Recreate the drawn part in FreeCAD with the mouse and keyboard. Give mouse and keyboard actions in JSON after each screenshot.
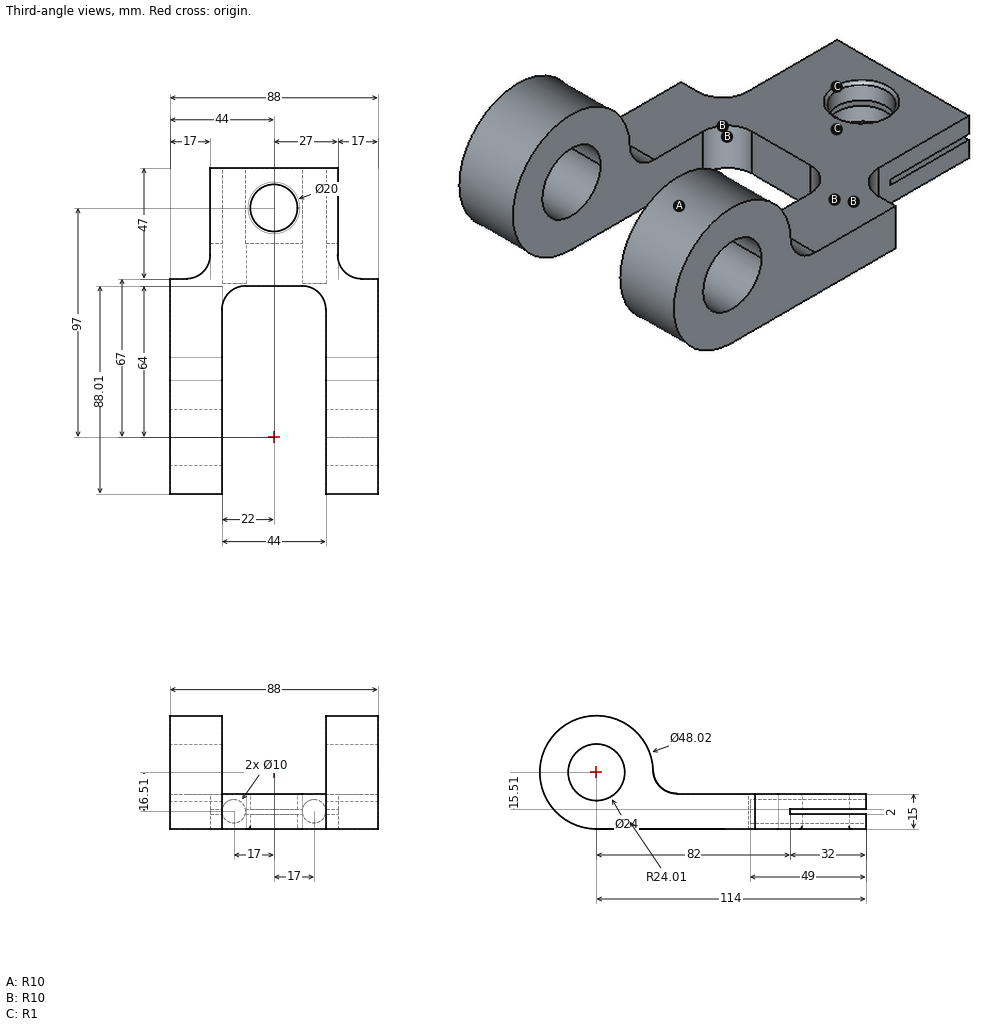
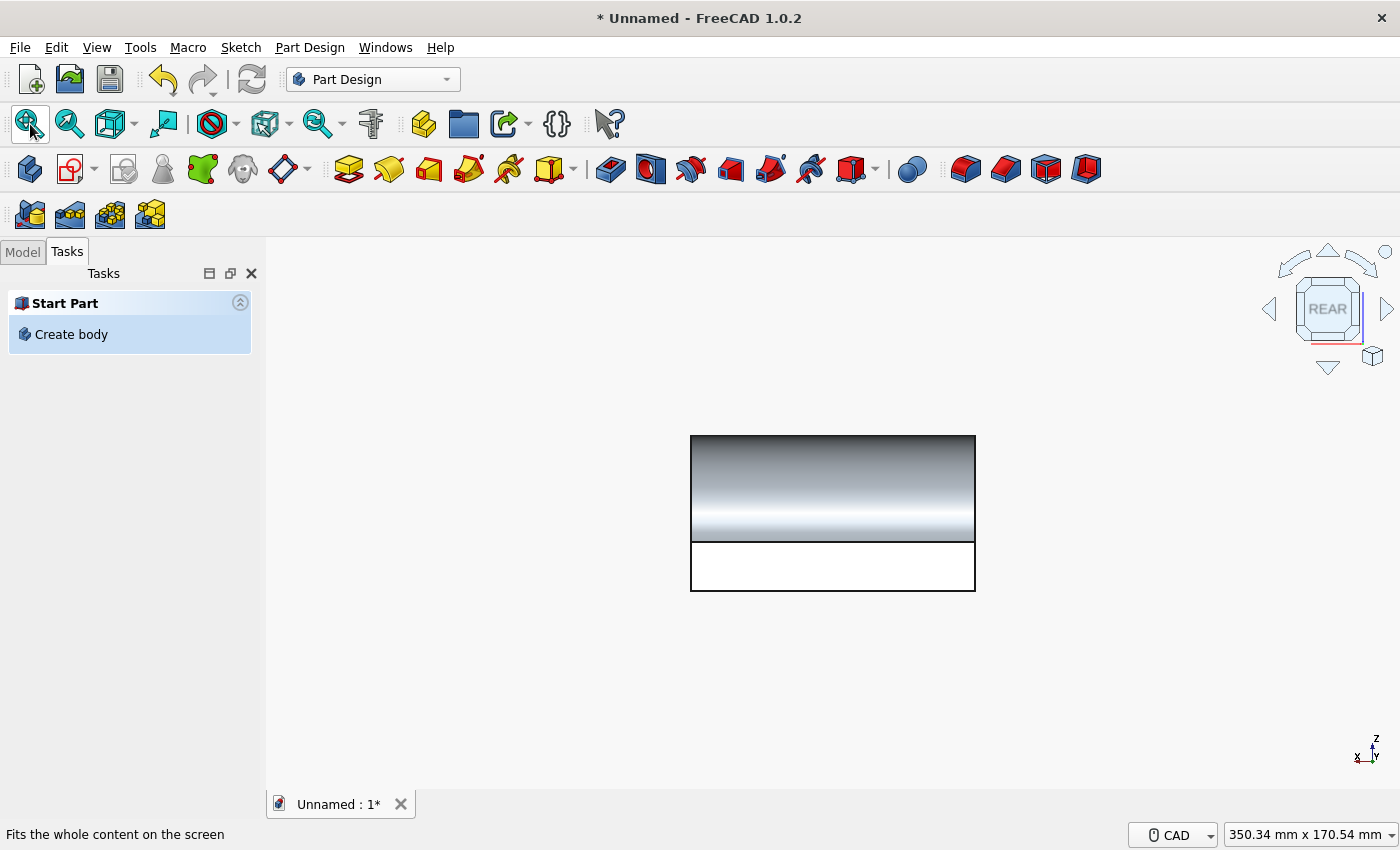
{"action": "key", "text": "6"}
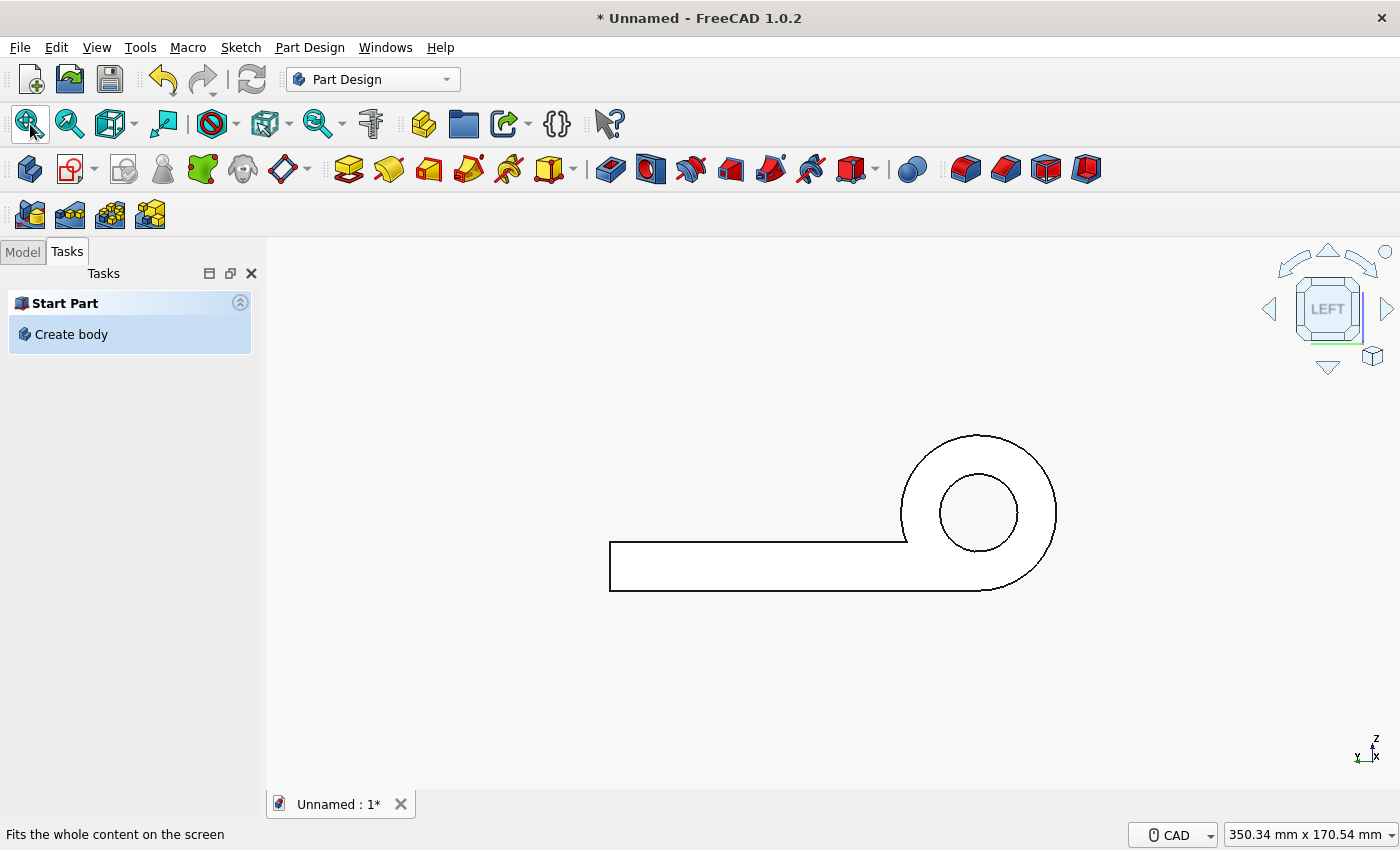
{"action": "left_click", "coordinate": [30, 124]}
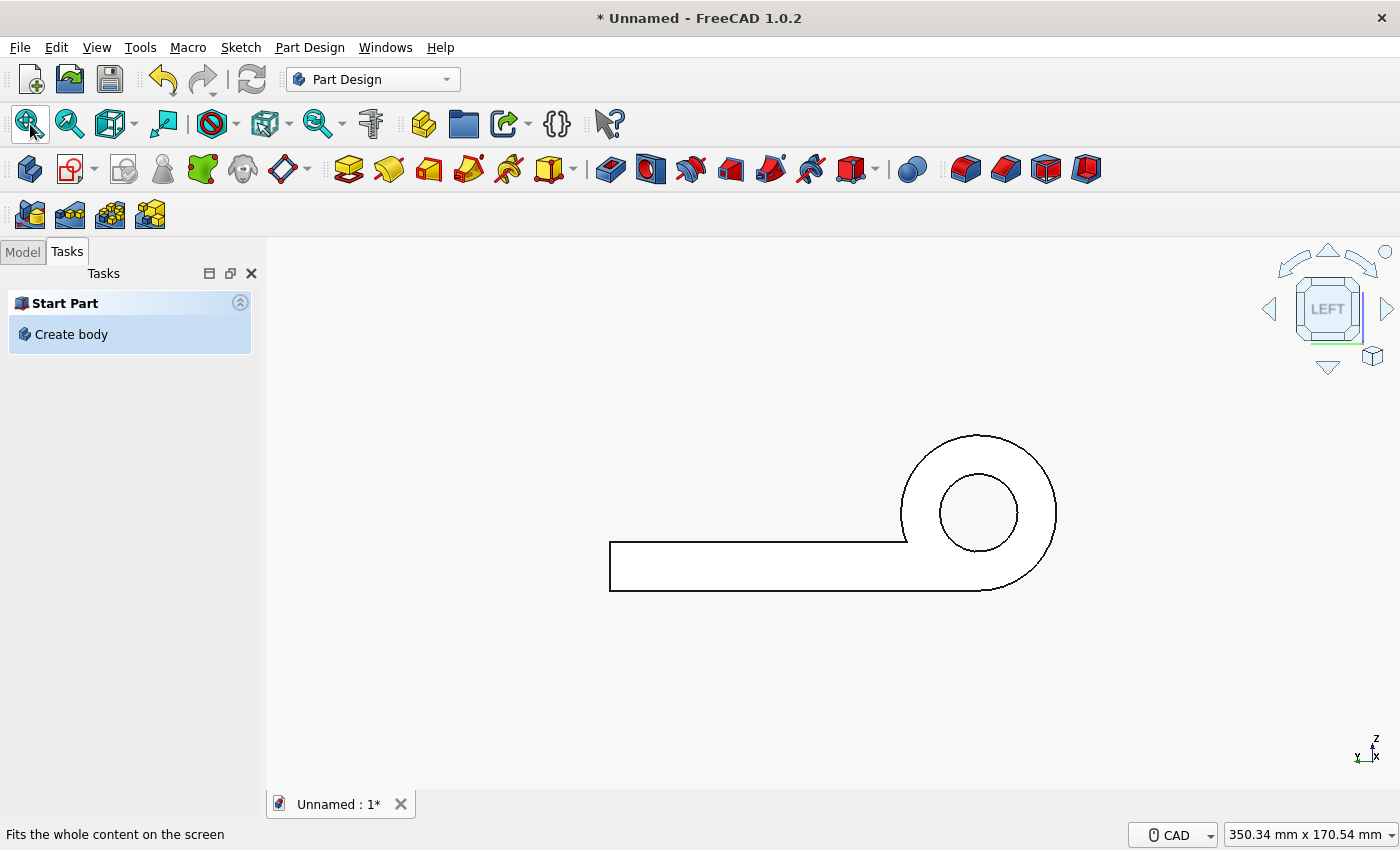
{"action": "key", "text": "v 3"}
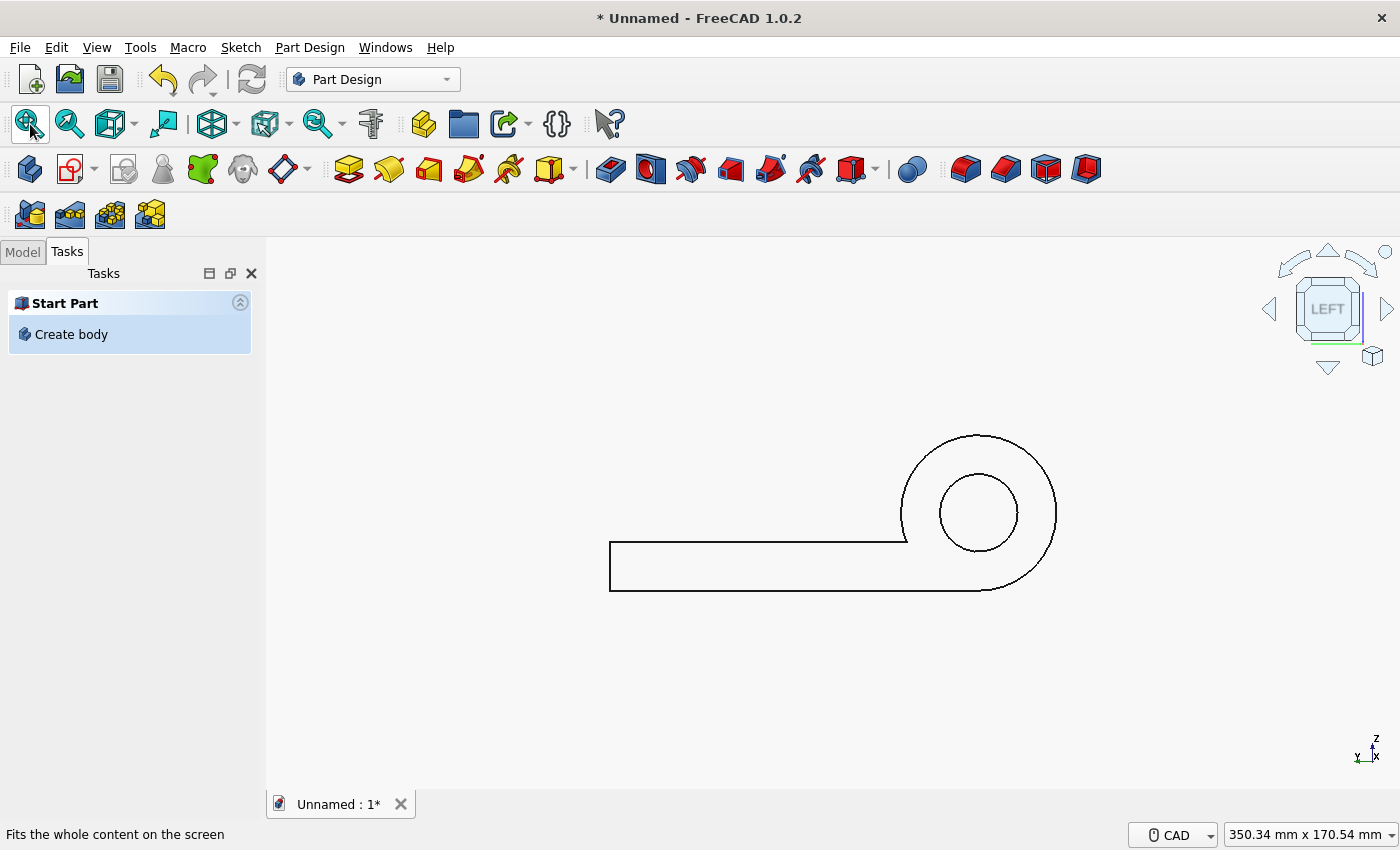
{"action": "key", "text": "0"}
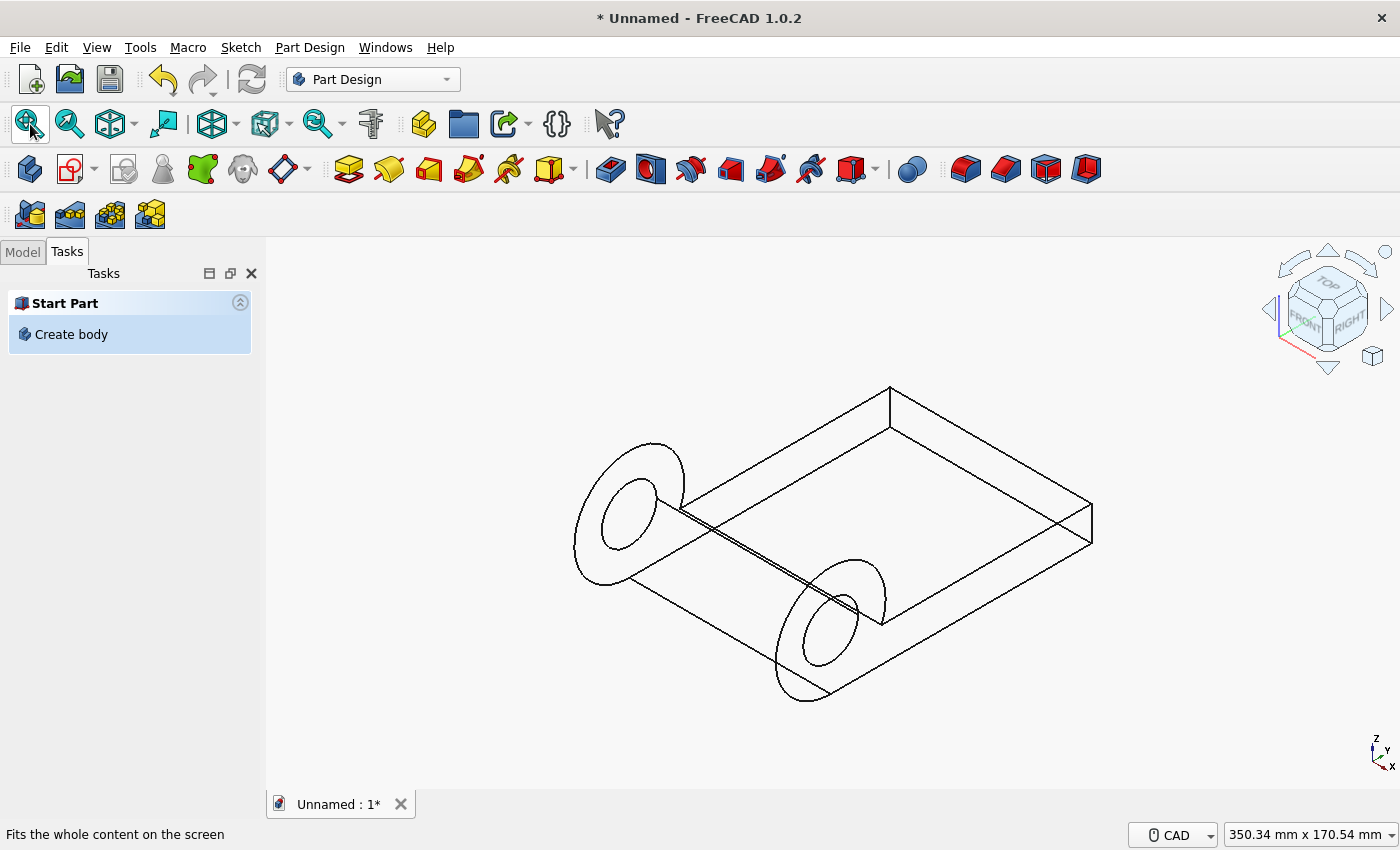
{"action": "key", "text": "2"}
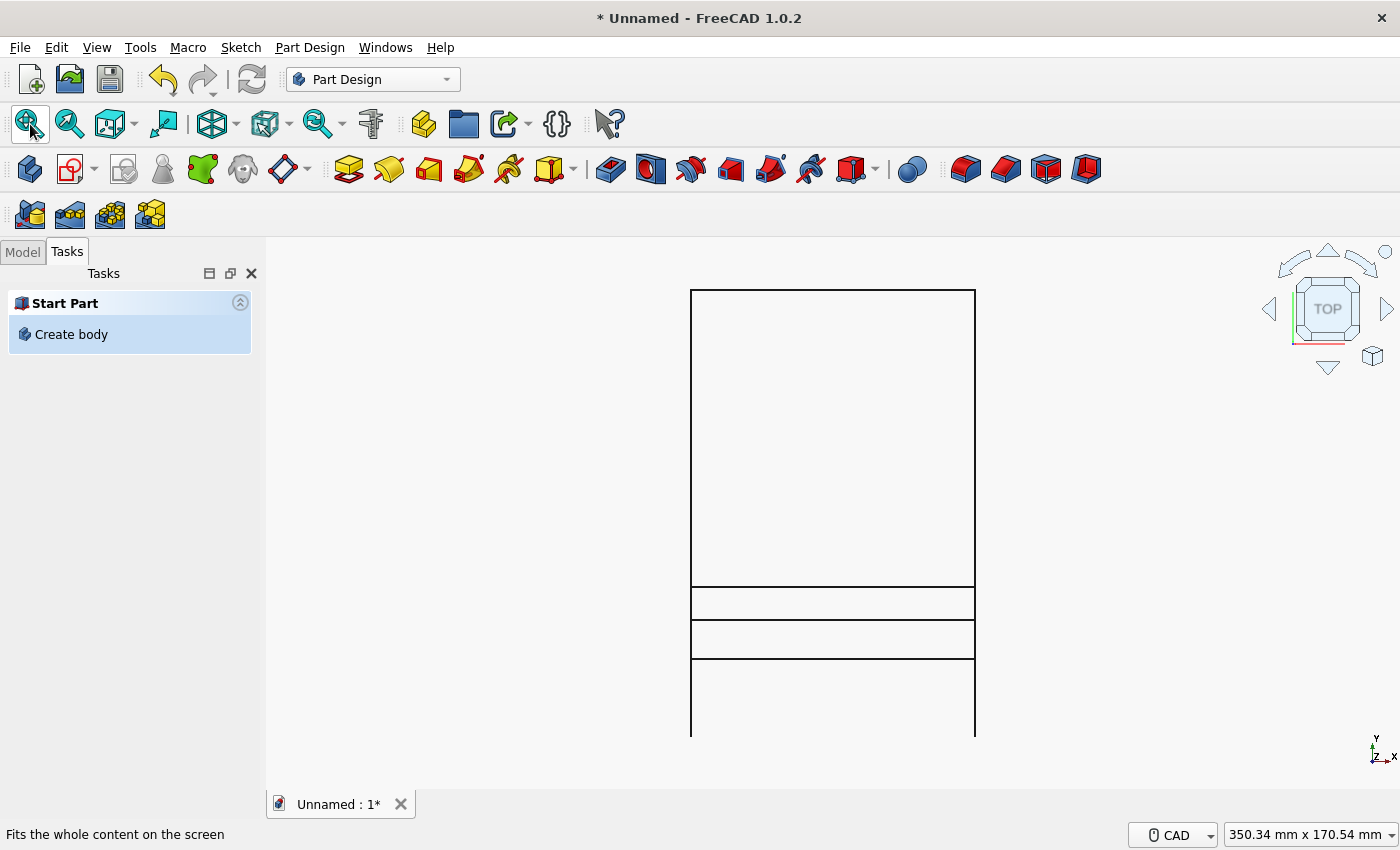
{"action": "left_click", "coordinate": [833, 586]}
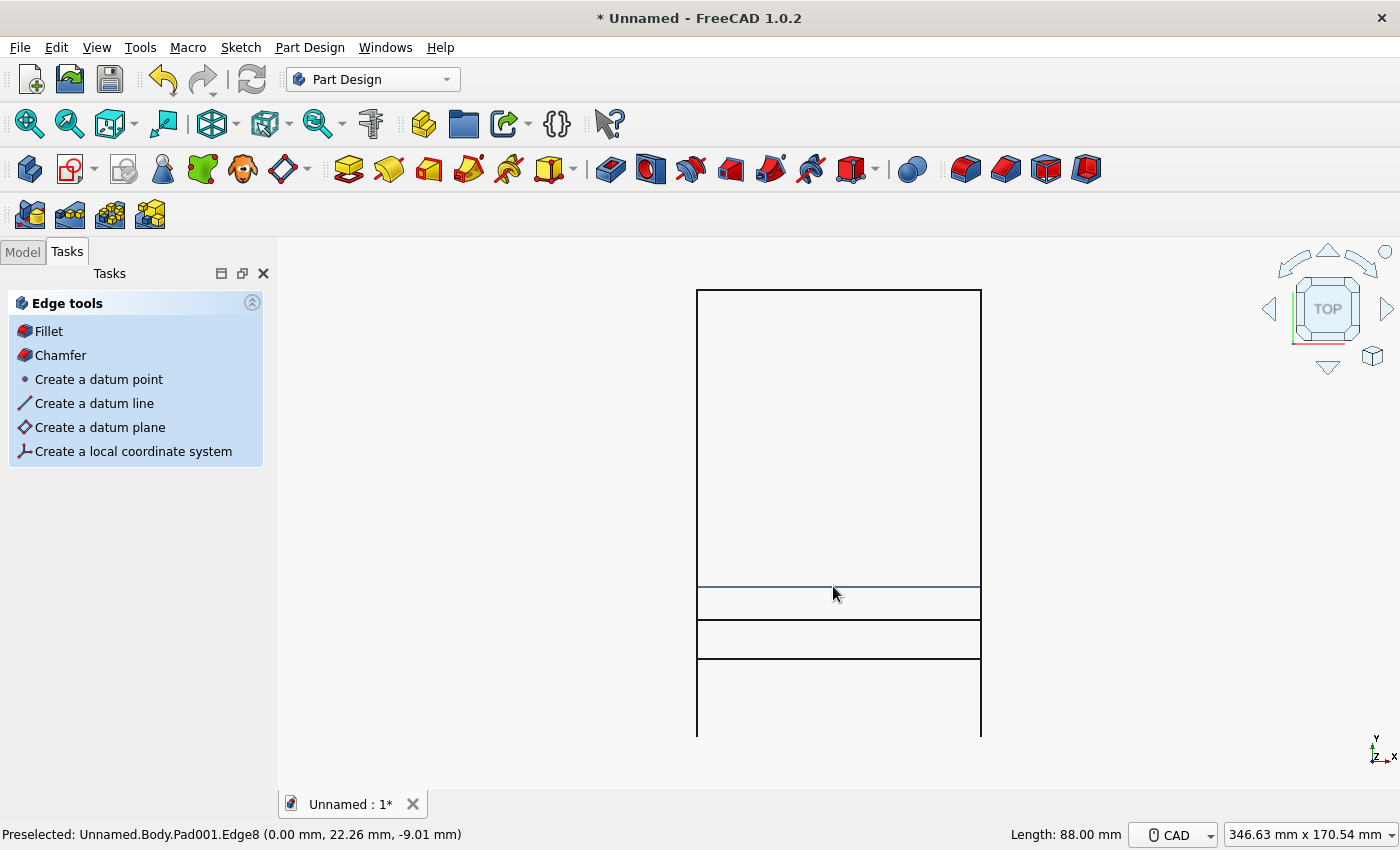
{"action": "key", "text": "v 1"}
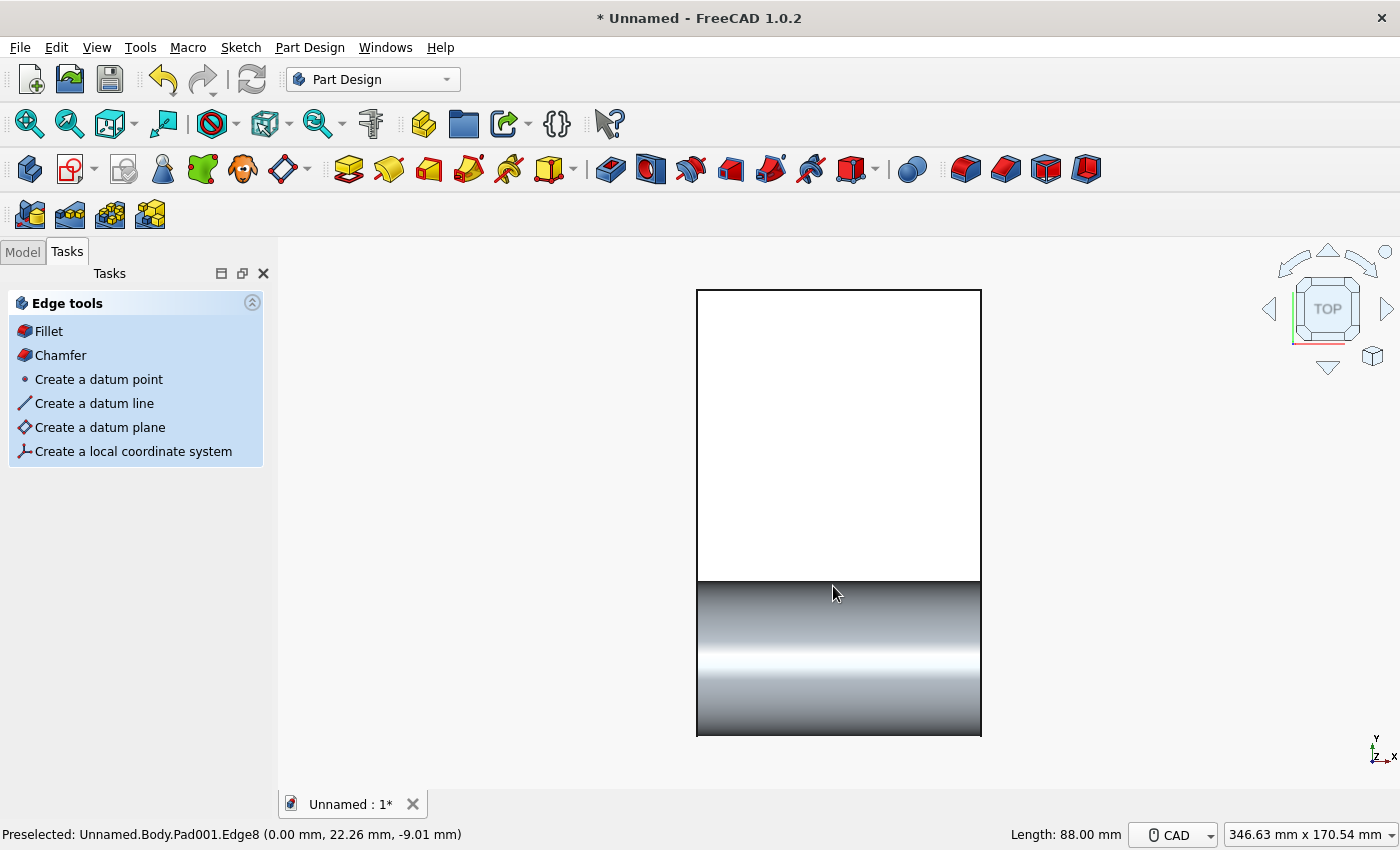
{"action": "left_click", "coordinate": [966, 170]}